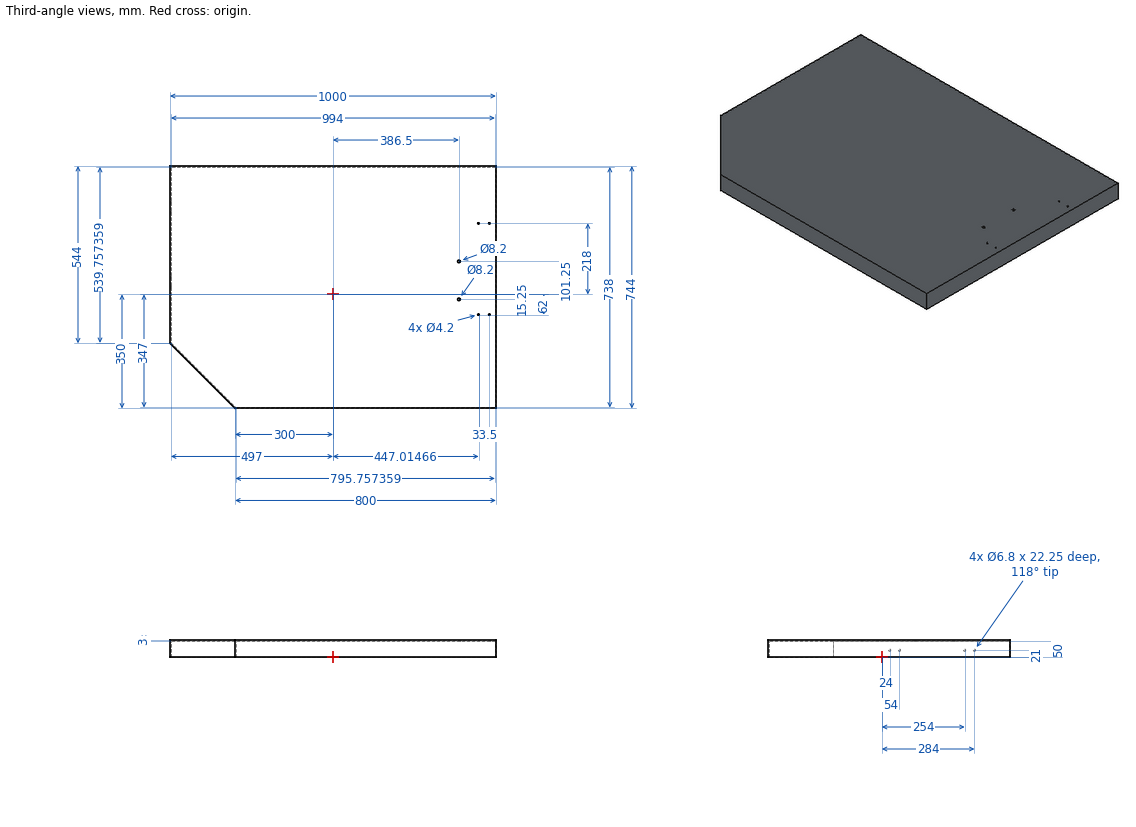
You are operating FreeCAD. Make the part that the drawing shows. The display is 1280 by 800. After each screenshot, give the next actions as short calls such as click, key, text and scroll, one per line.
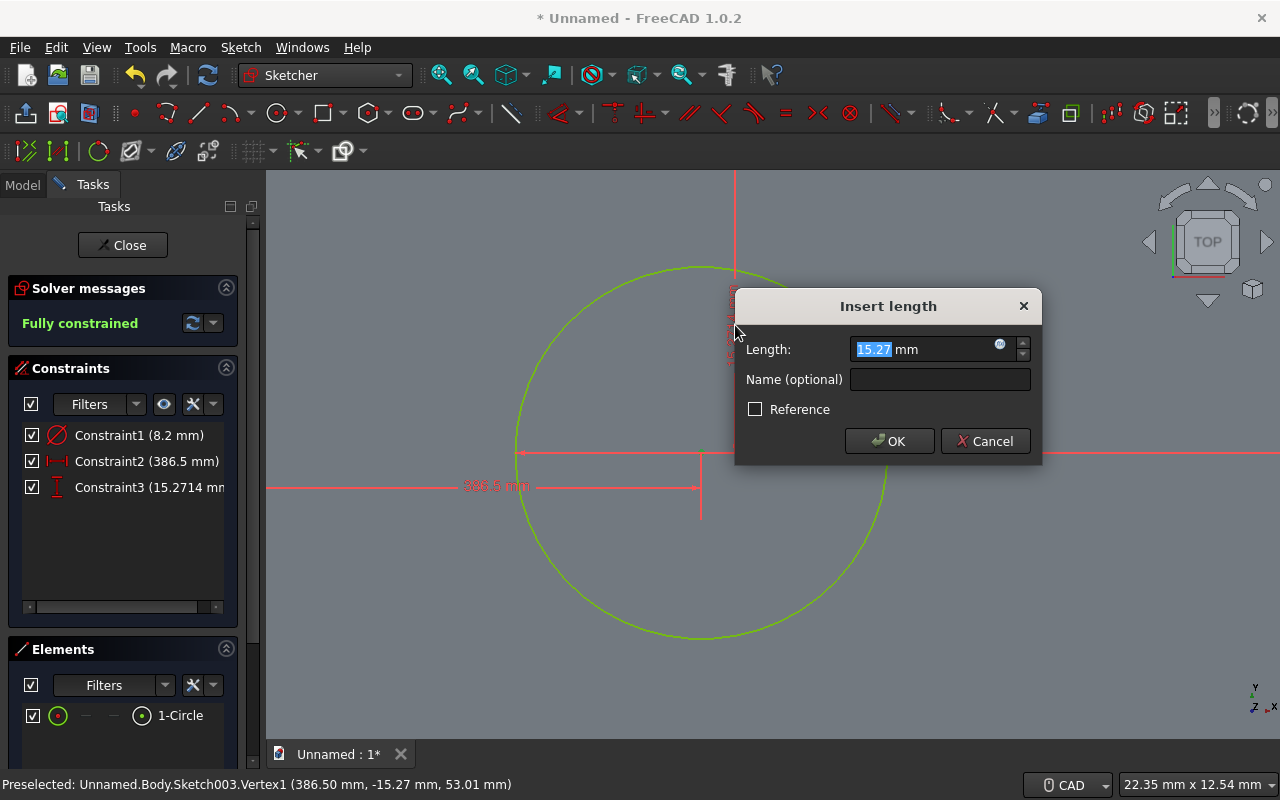
text(15.25)
key(Return)
key(Escape)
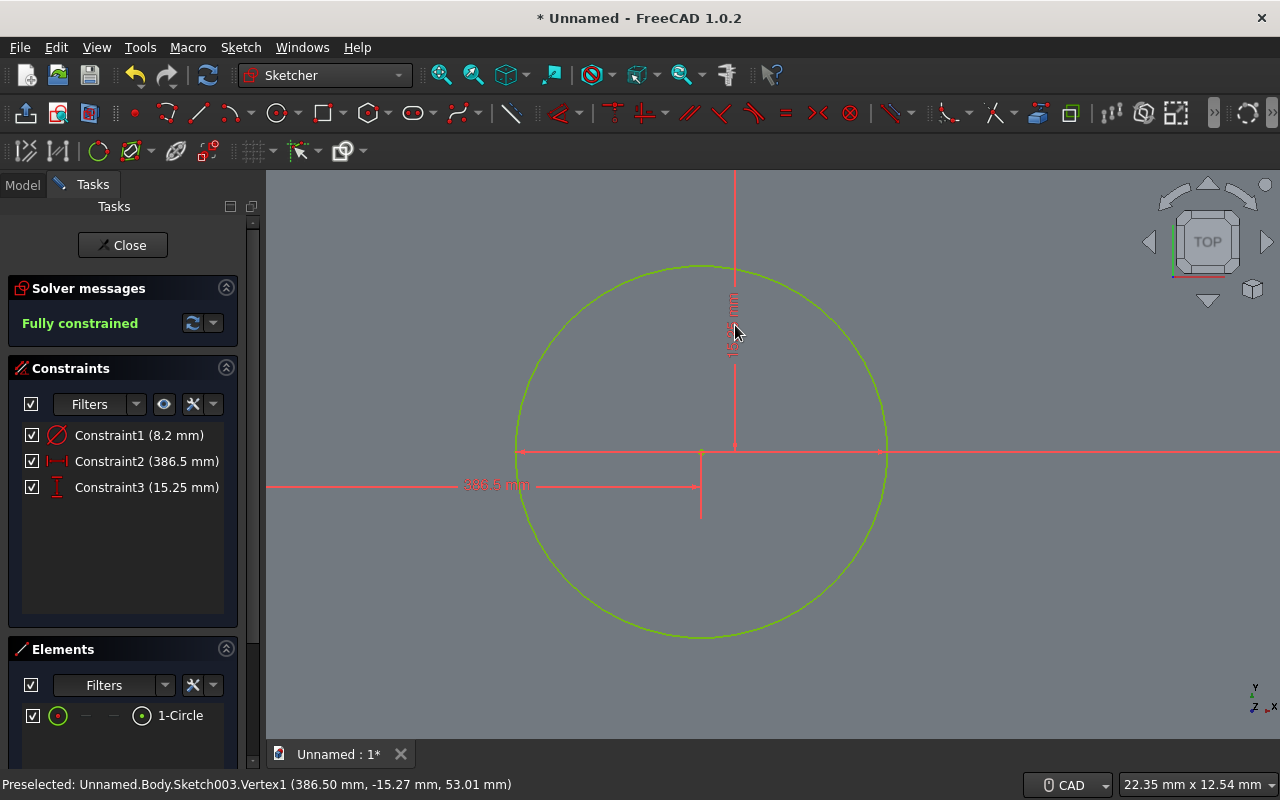
click(123, 245)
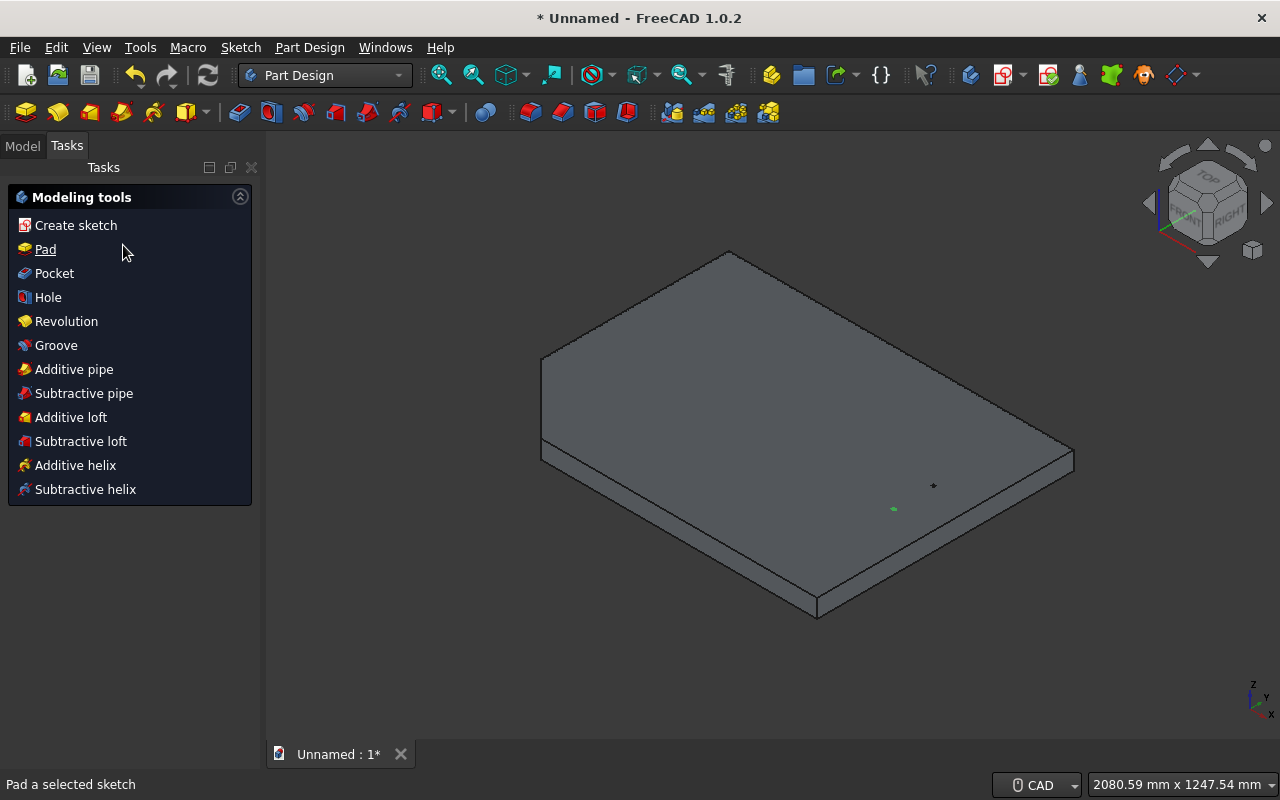
click(240, 112)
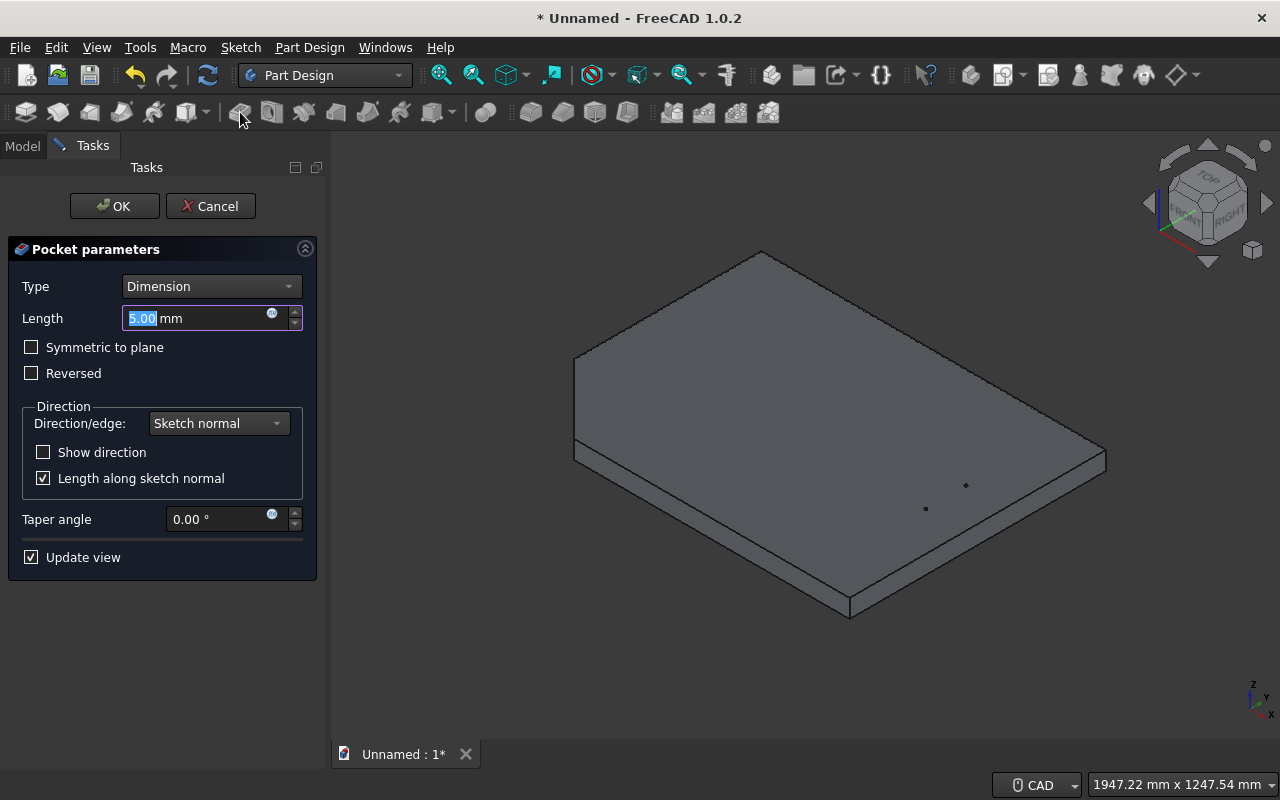
click(212, 286)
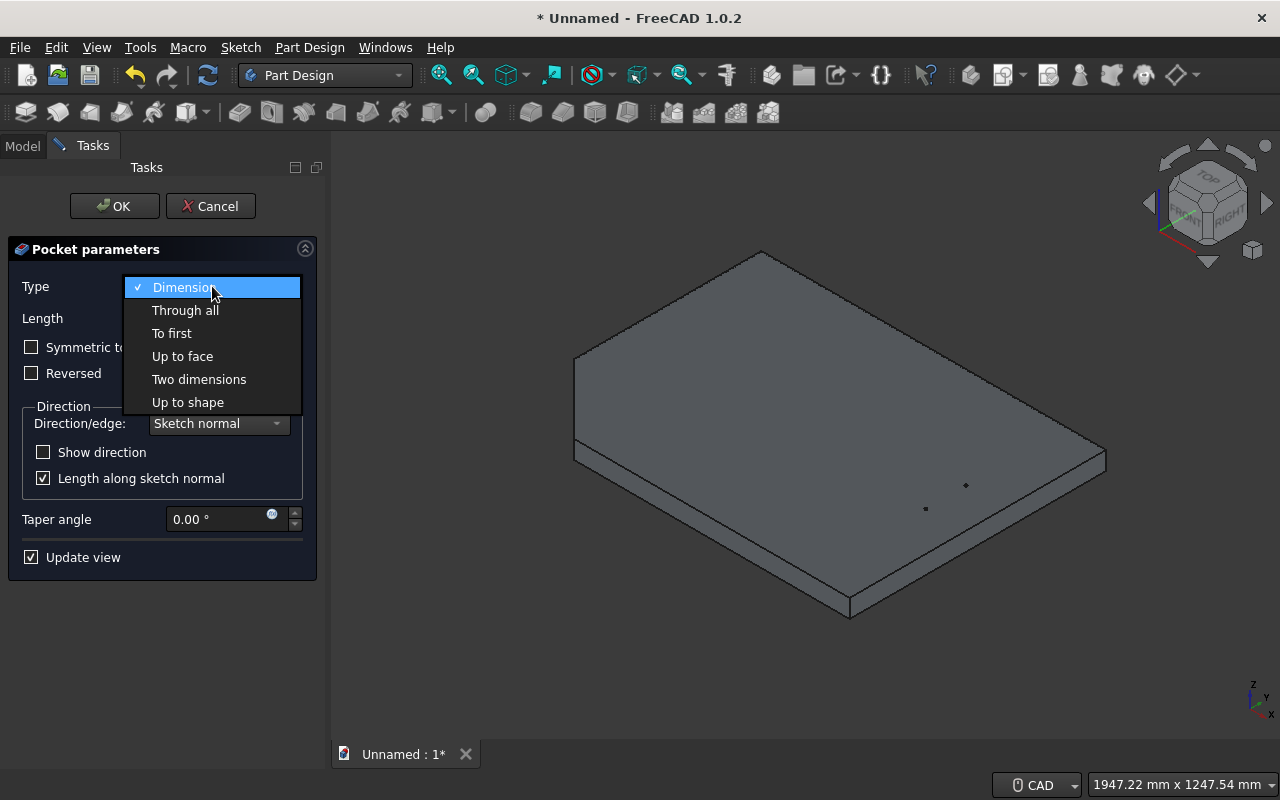
click(212, 334)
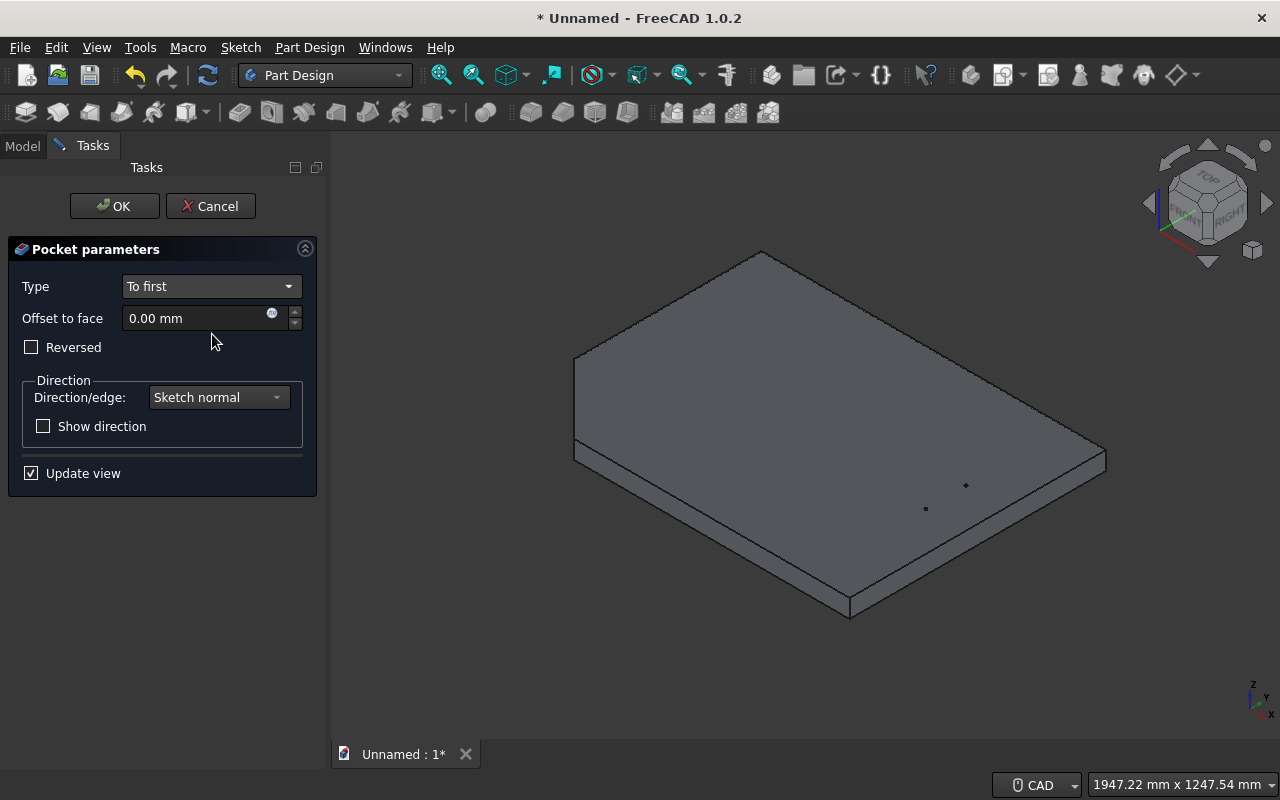
click(115, 206)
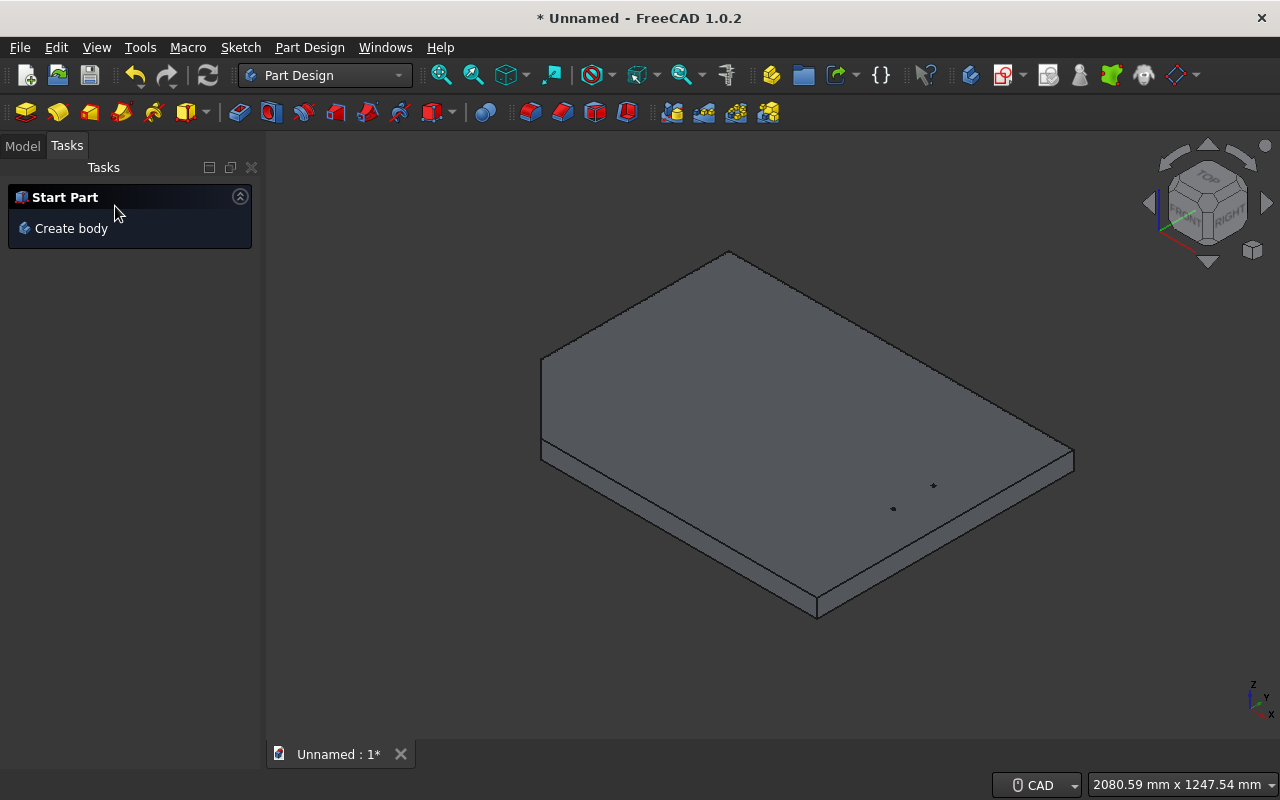
key(6)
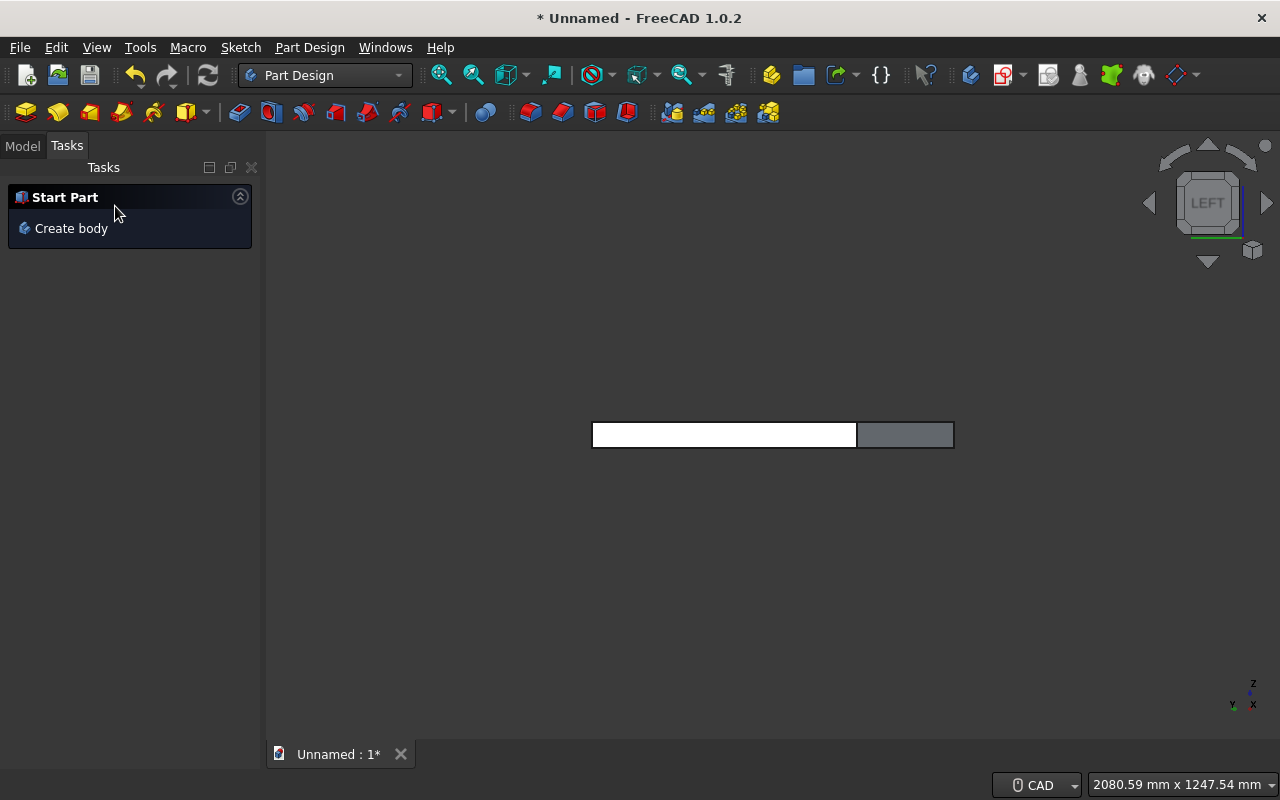
key(v)
key(f)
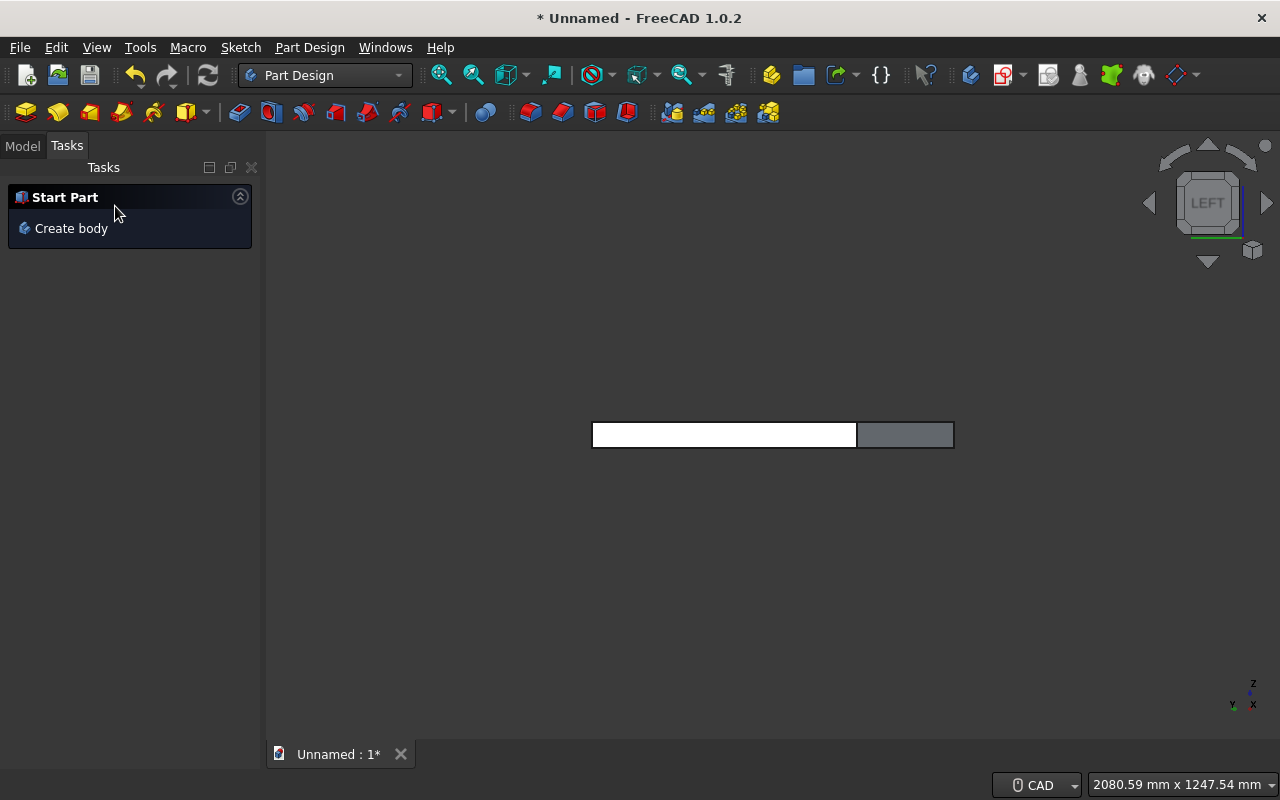
click(611, 434)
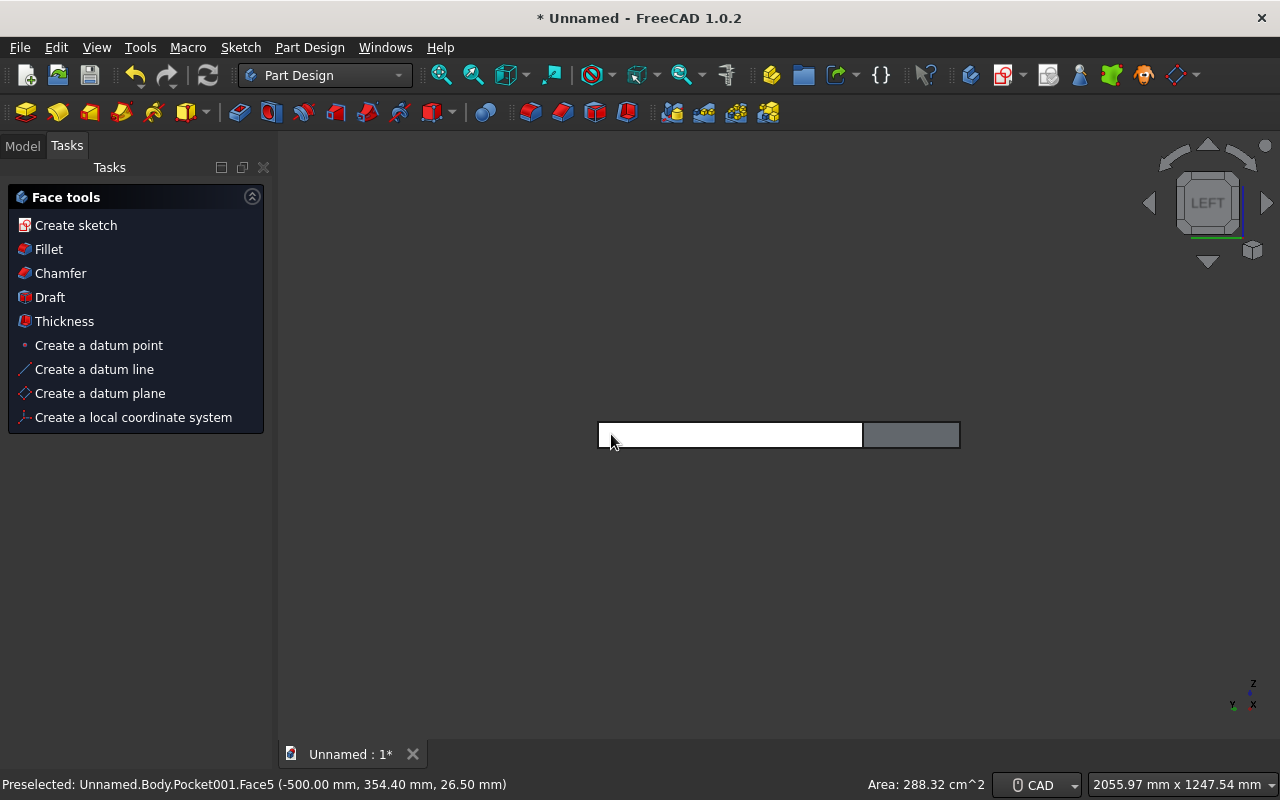
click(1004, 76)